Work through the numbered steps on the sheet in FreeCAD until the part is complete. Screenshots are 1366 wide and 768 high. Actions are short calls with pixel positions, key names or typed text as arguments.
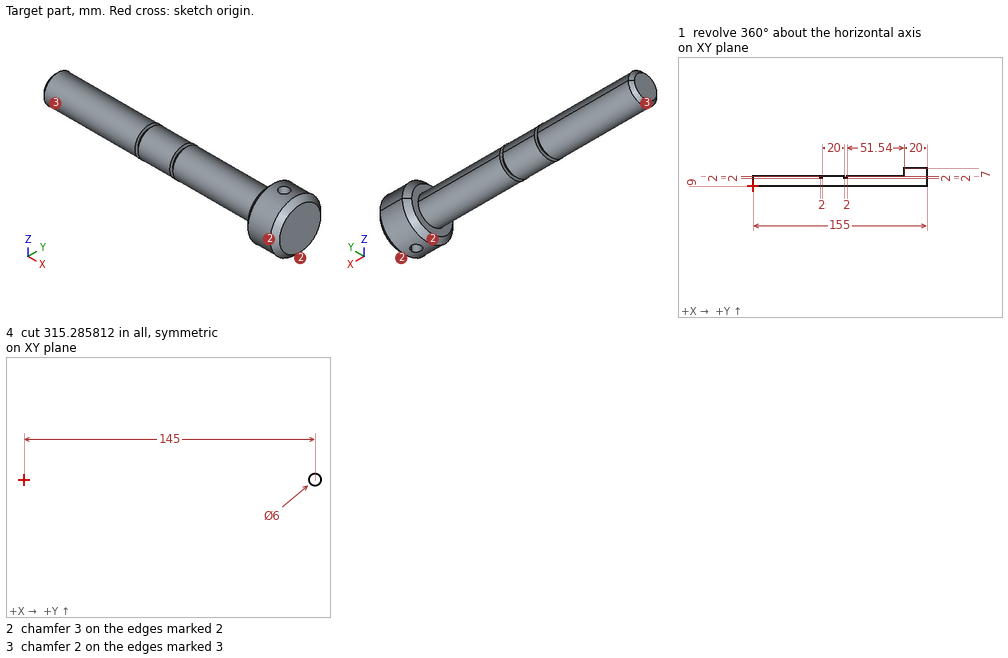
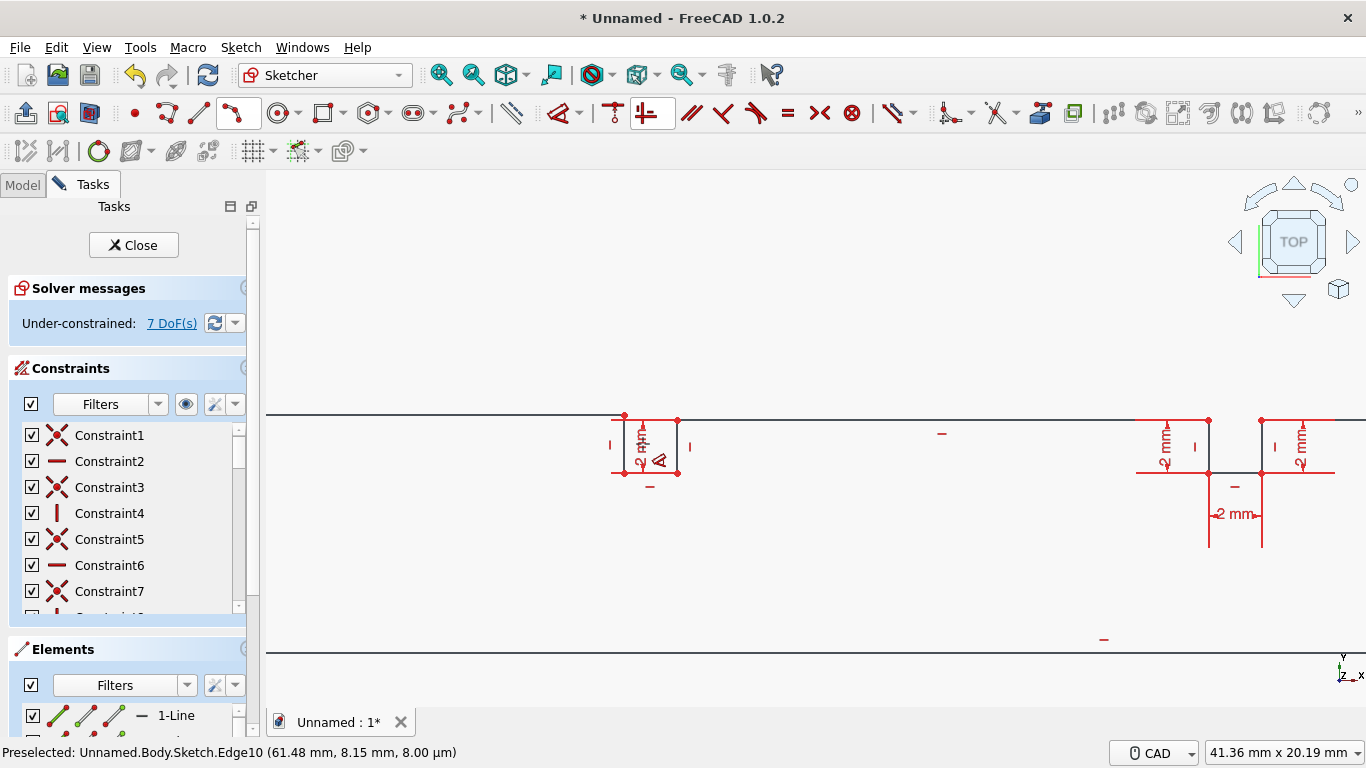
click(661, 473)
click(651, 507)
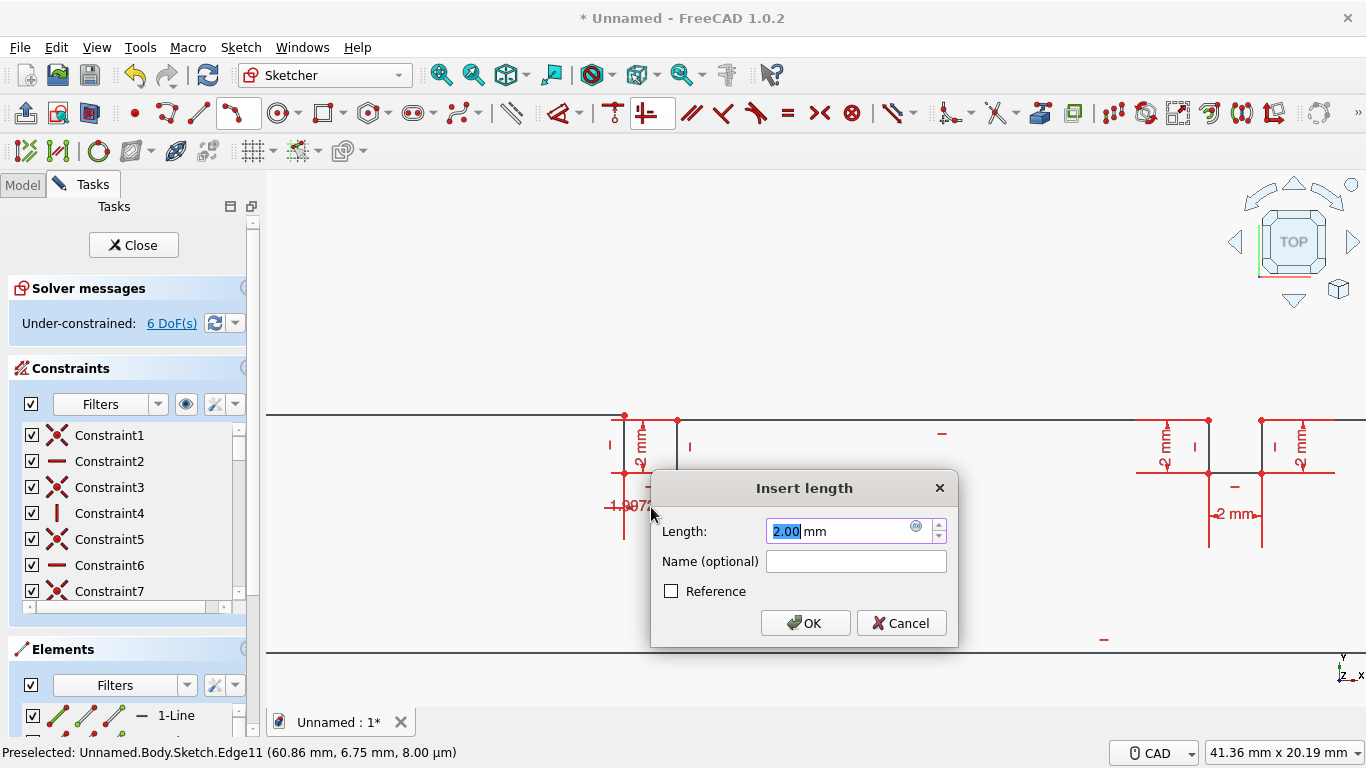
text(2)
key(Return)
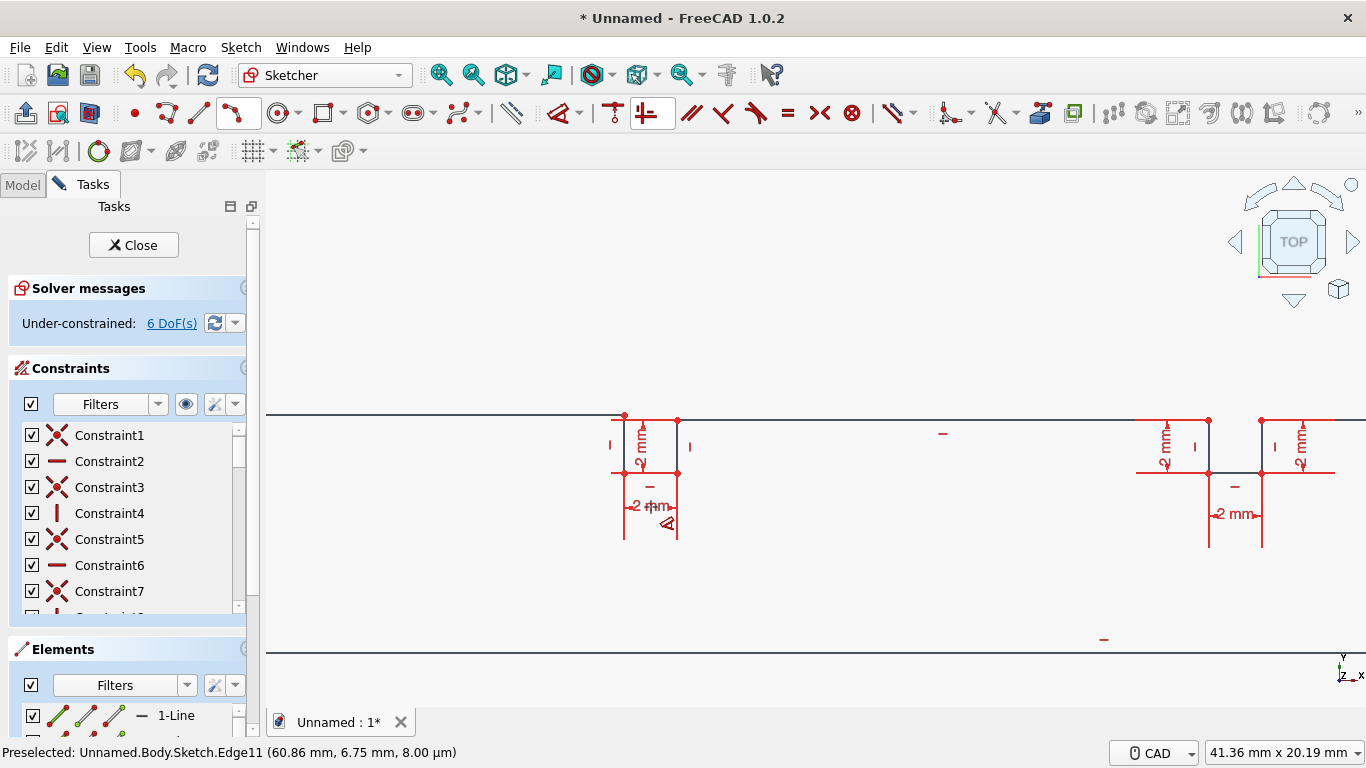
click(624, 456)
click(590, 465)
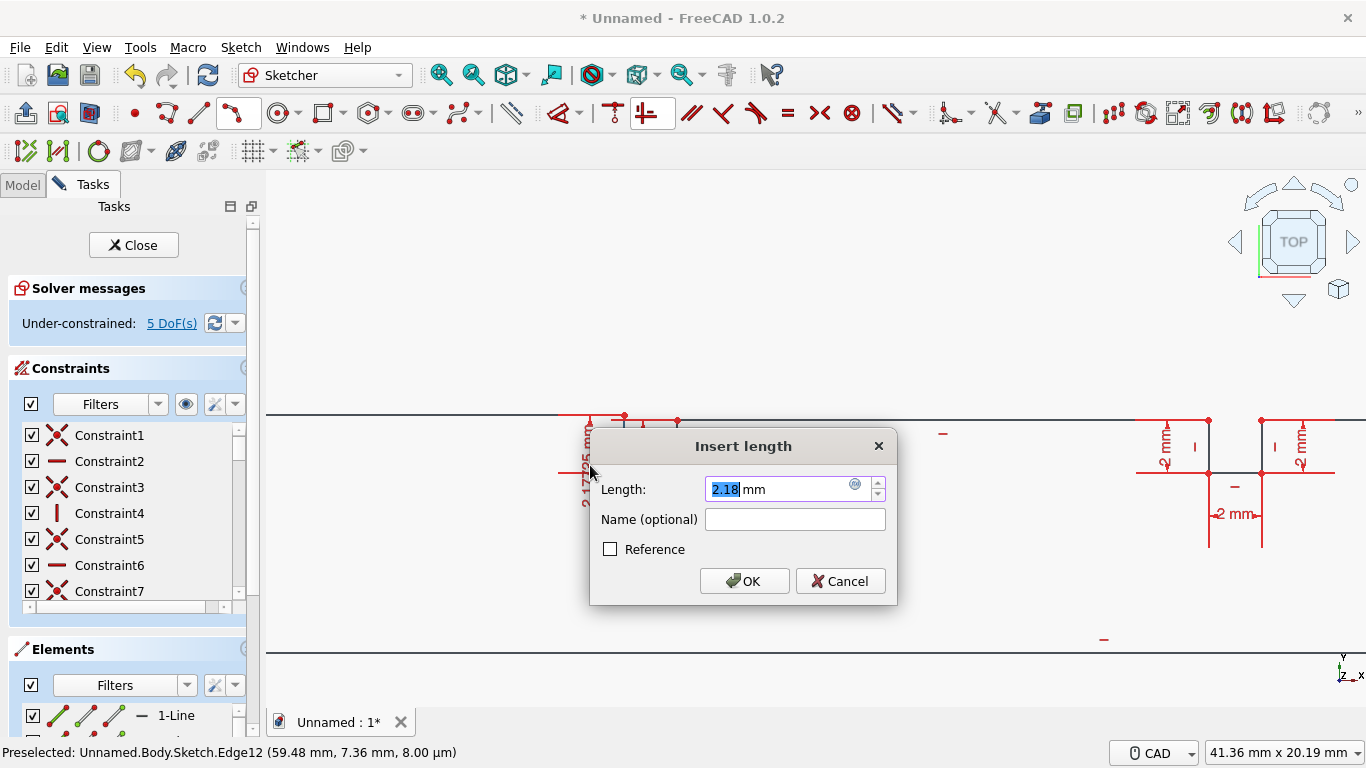
text(2)
key(Return)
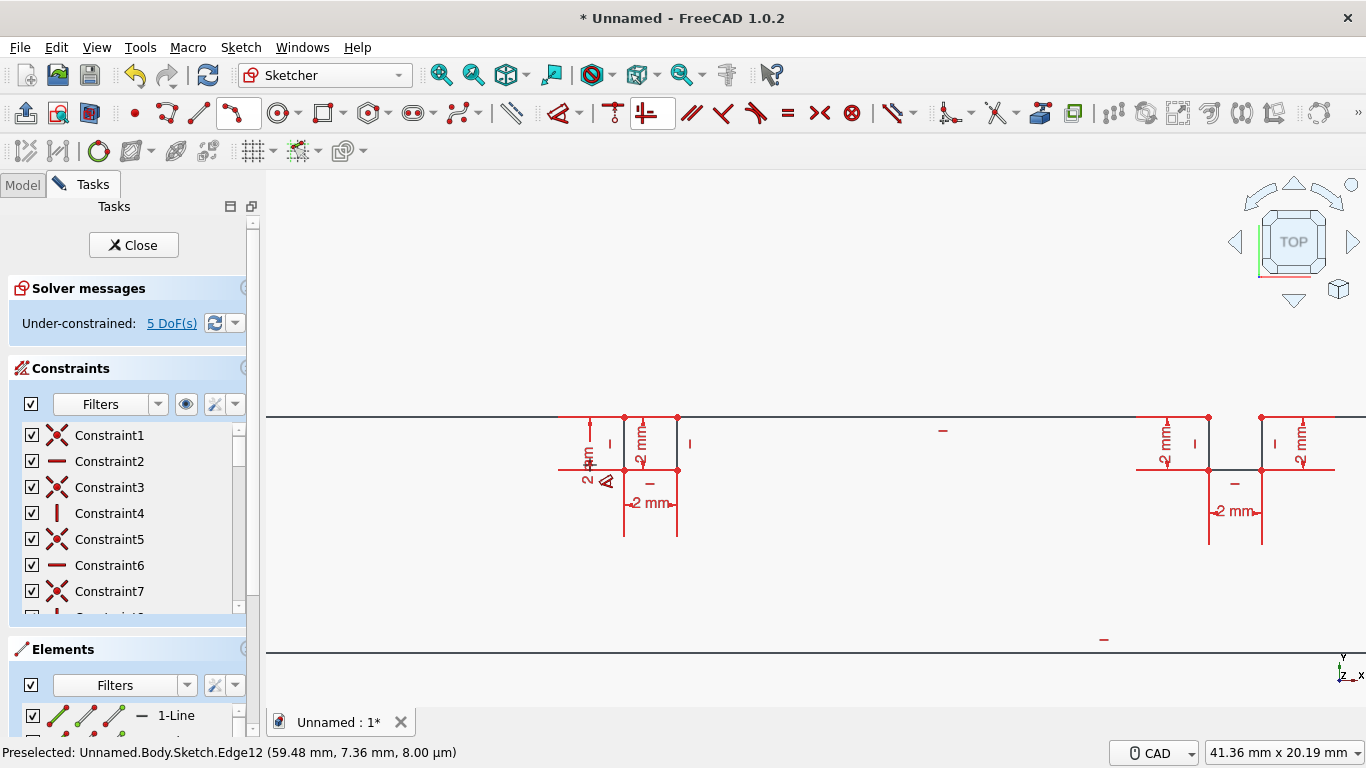
scroll(677, 438, down, 9)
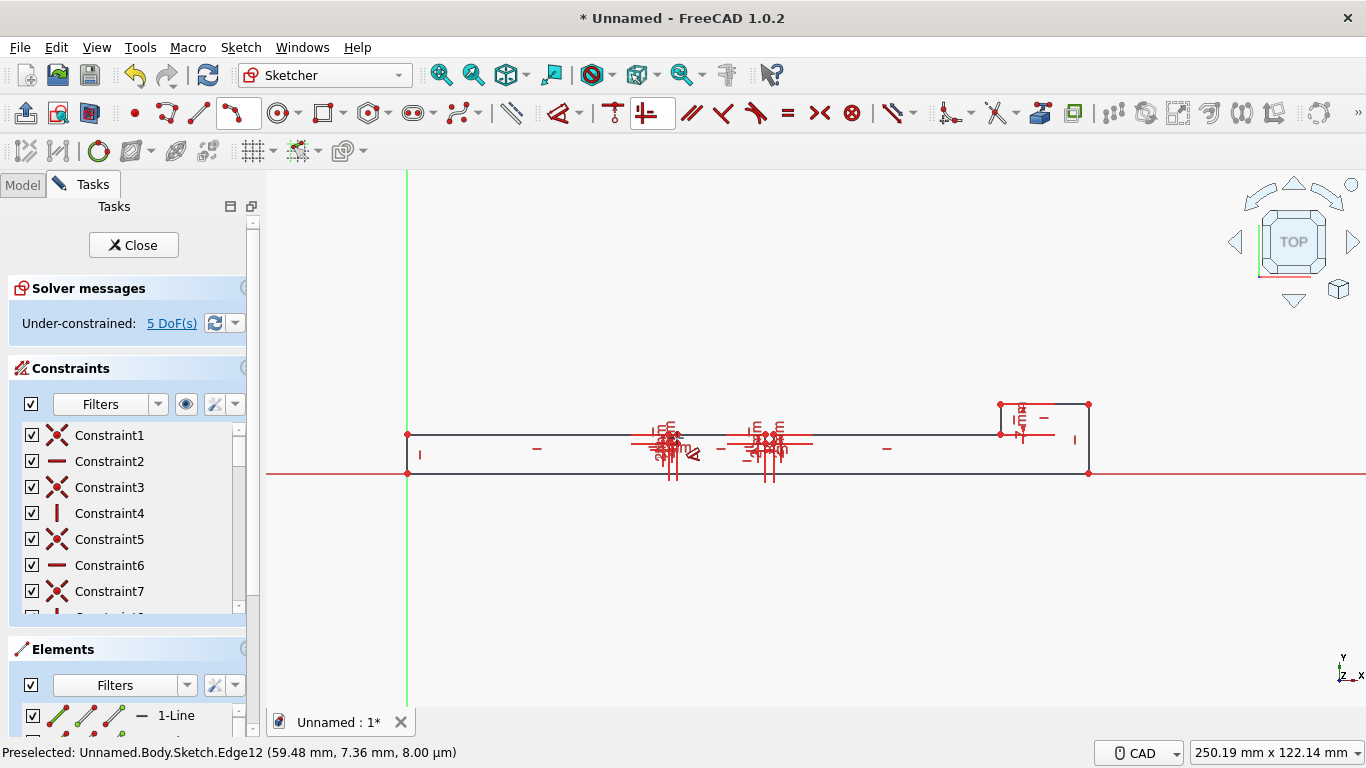
click(407, 447)
click(373, 454)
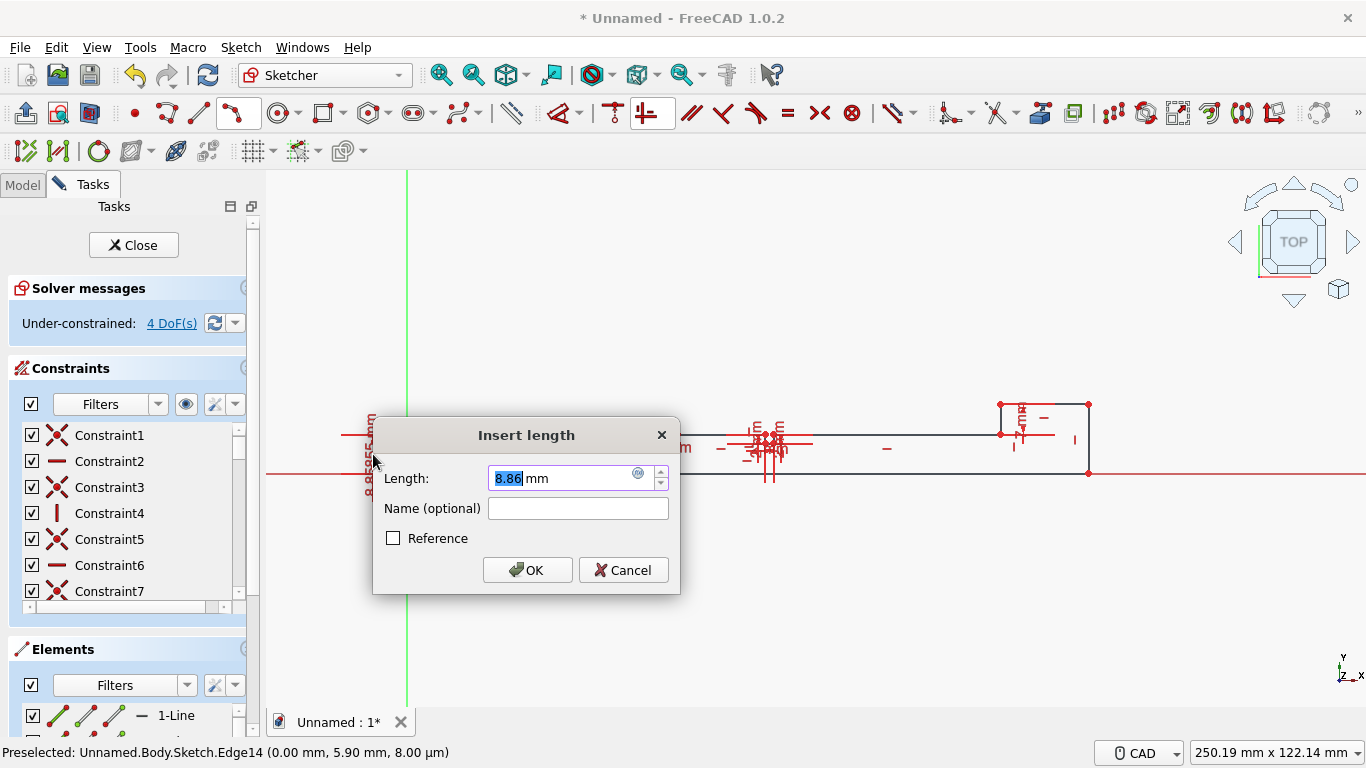
text(9)
key(Return)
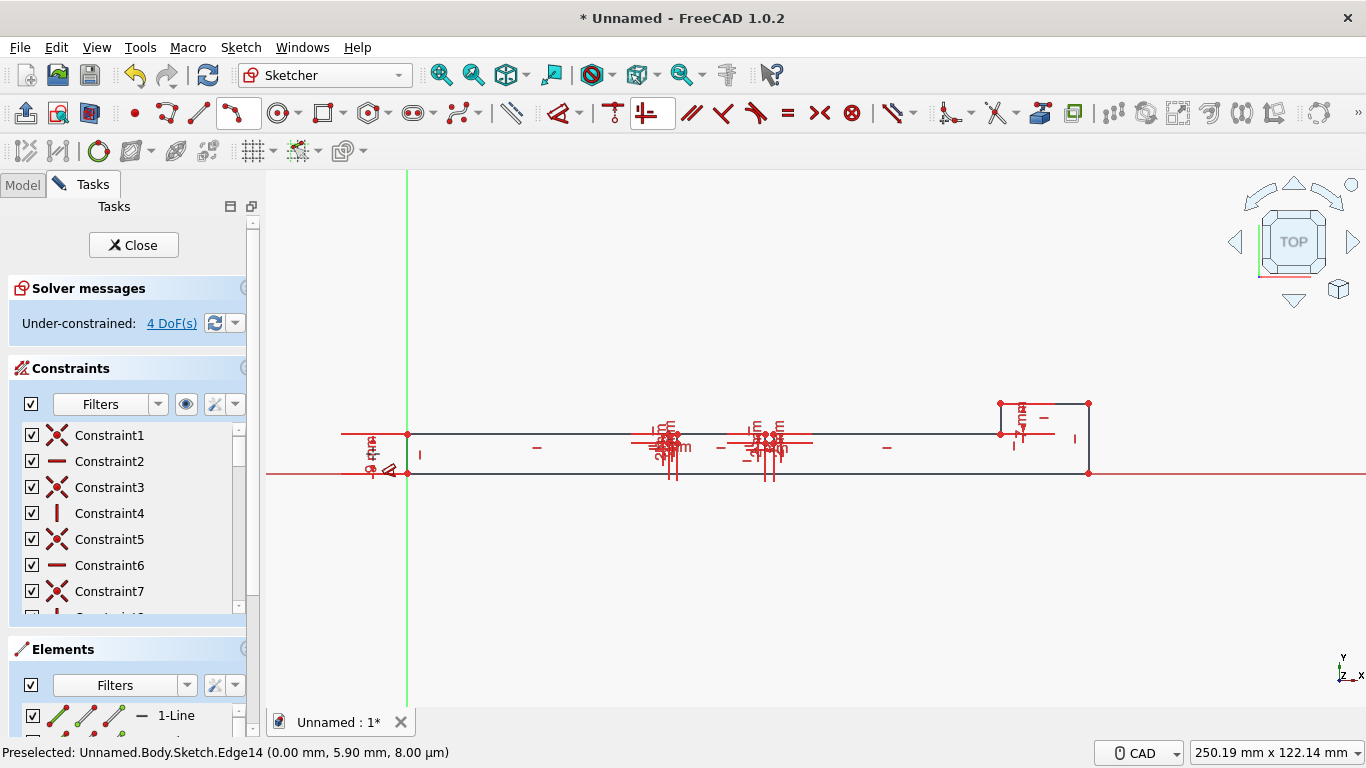
click(1062, 404)
click(1045, 370)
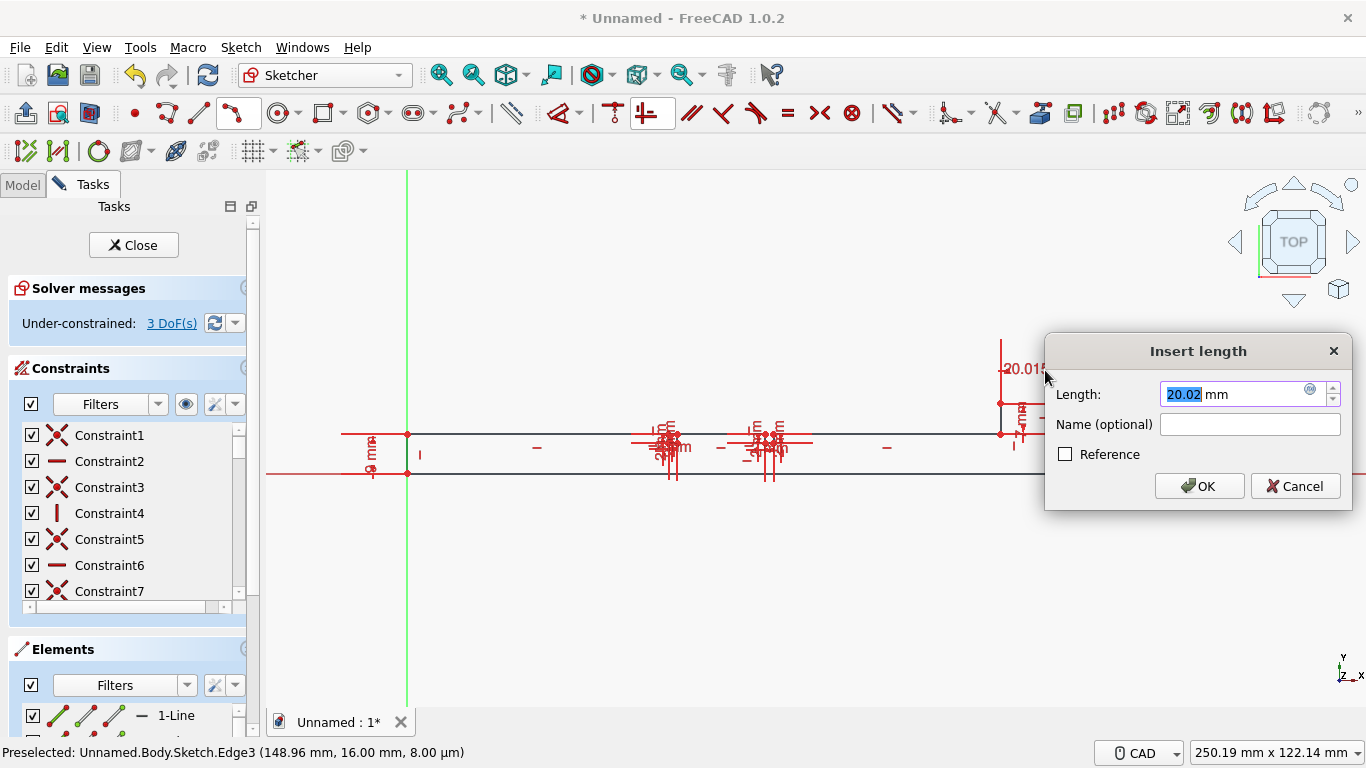
text(20)
key(Return)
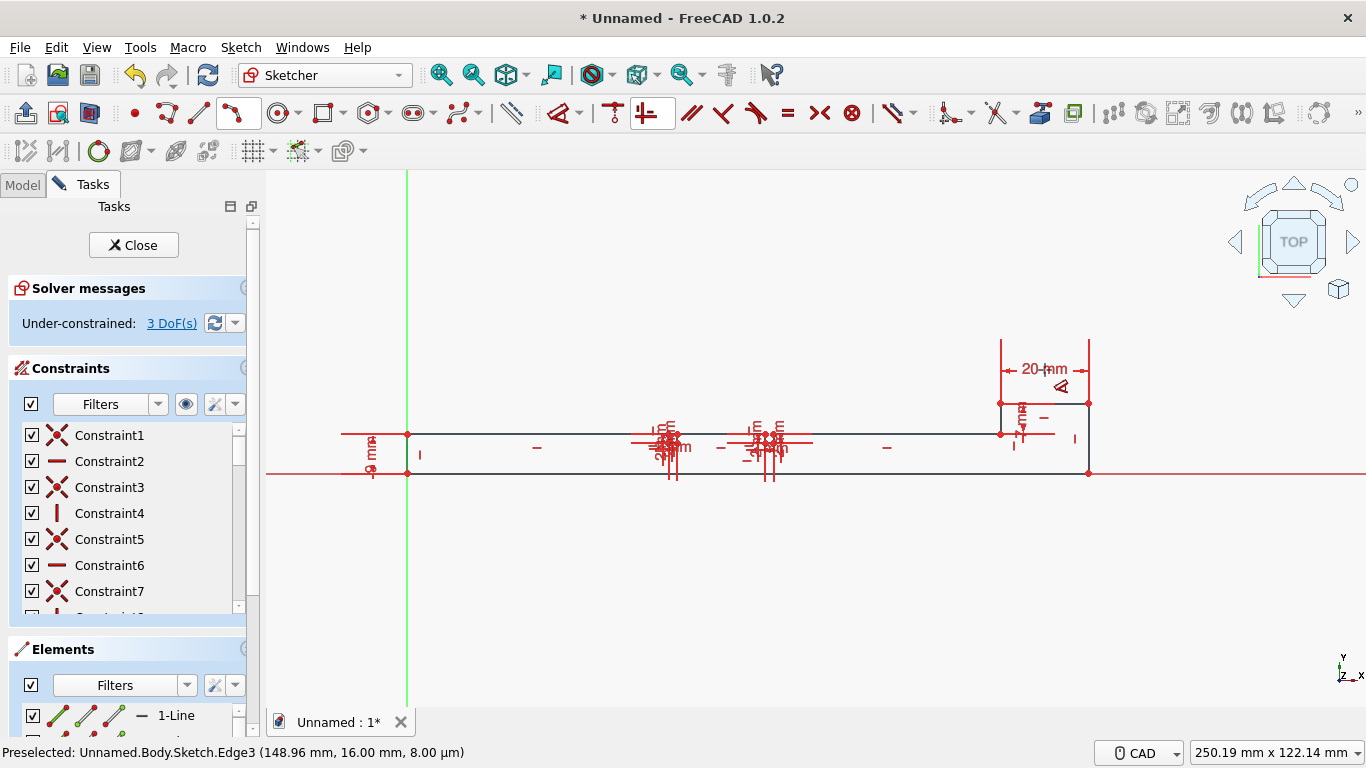
click(739, 434)
click(721, 400)